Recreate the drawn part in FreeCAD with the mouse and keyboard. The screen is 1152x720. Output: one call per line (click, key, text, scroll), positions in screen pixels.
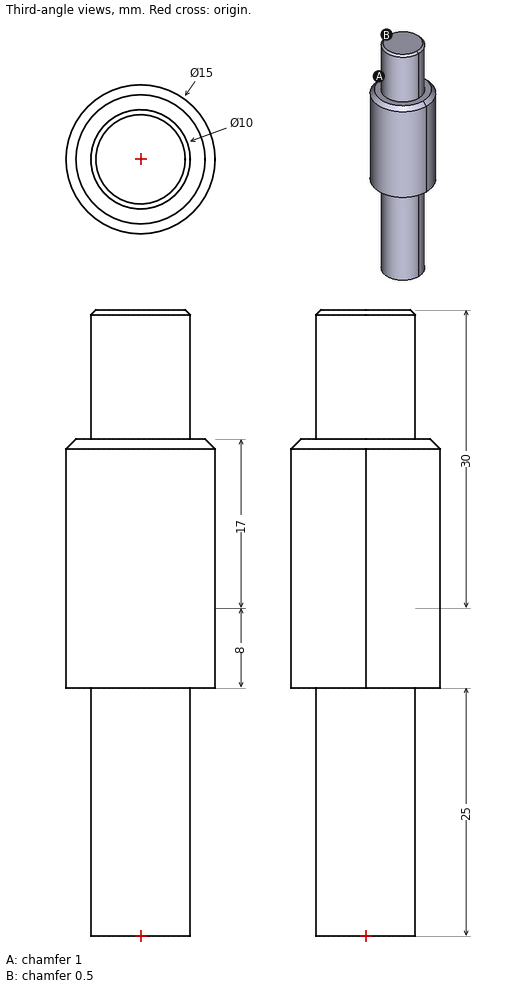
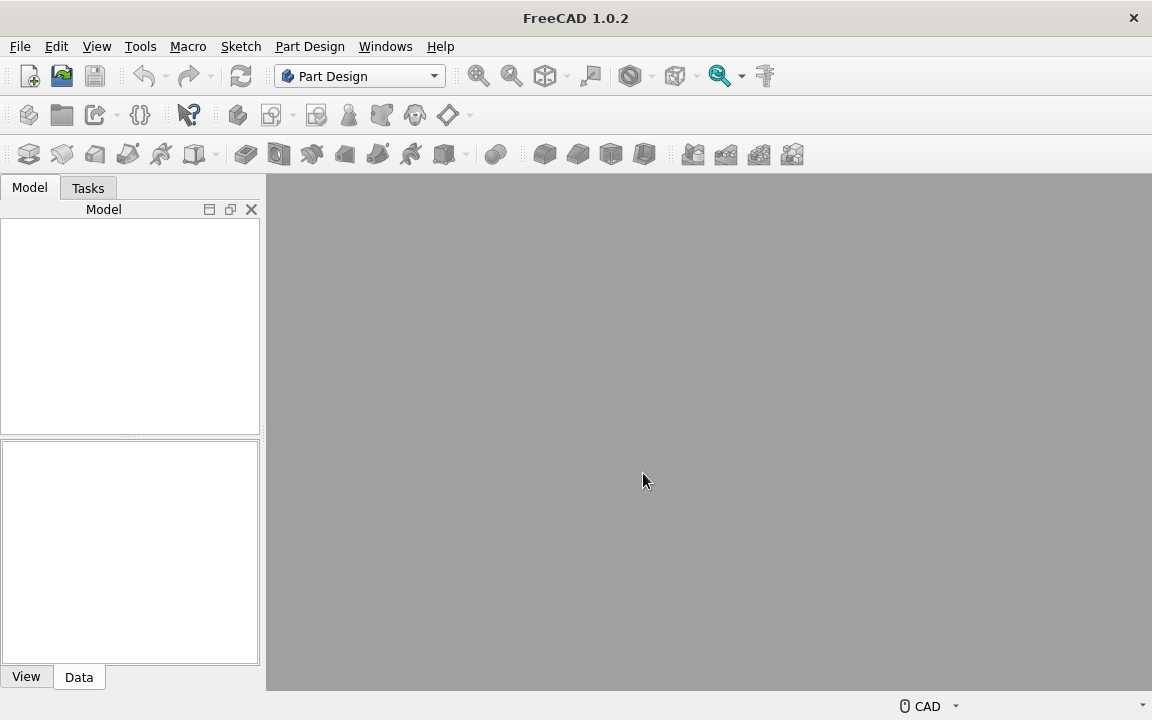
key(ctrl+n)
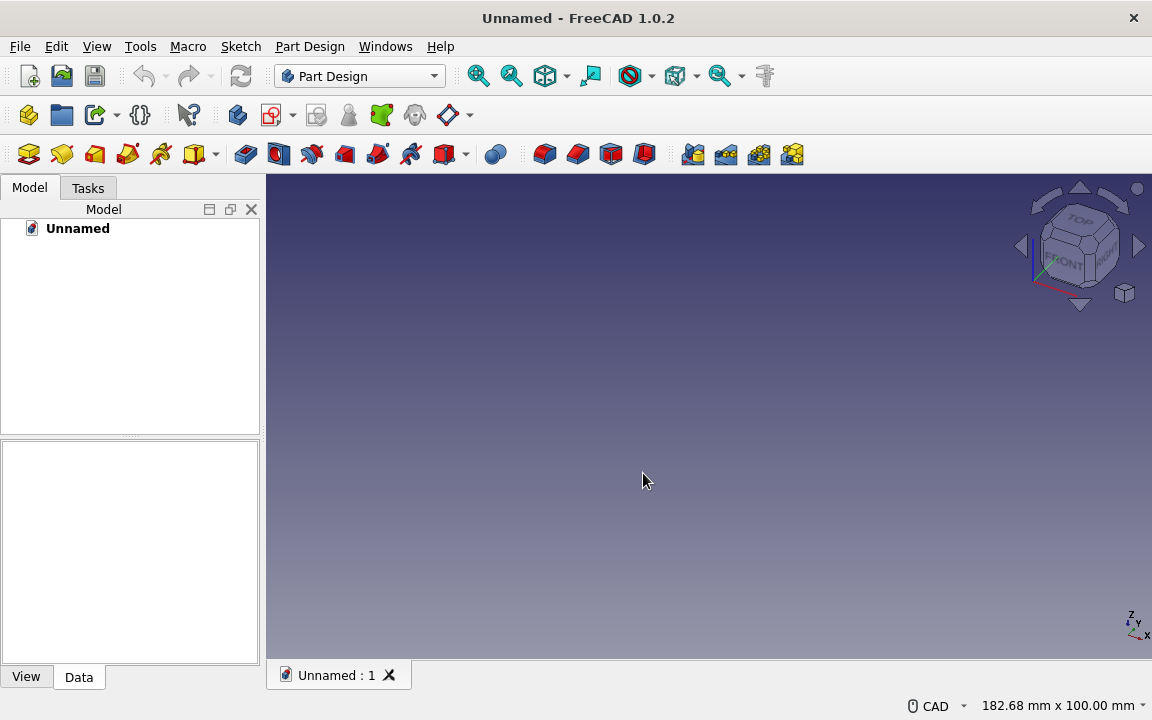
click(270, 116)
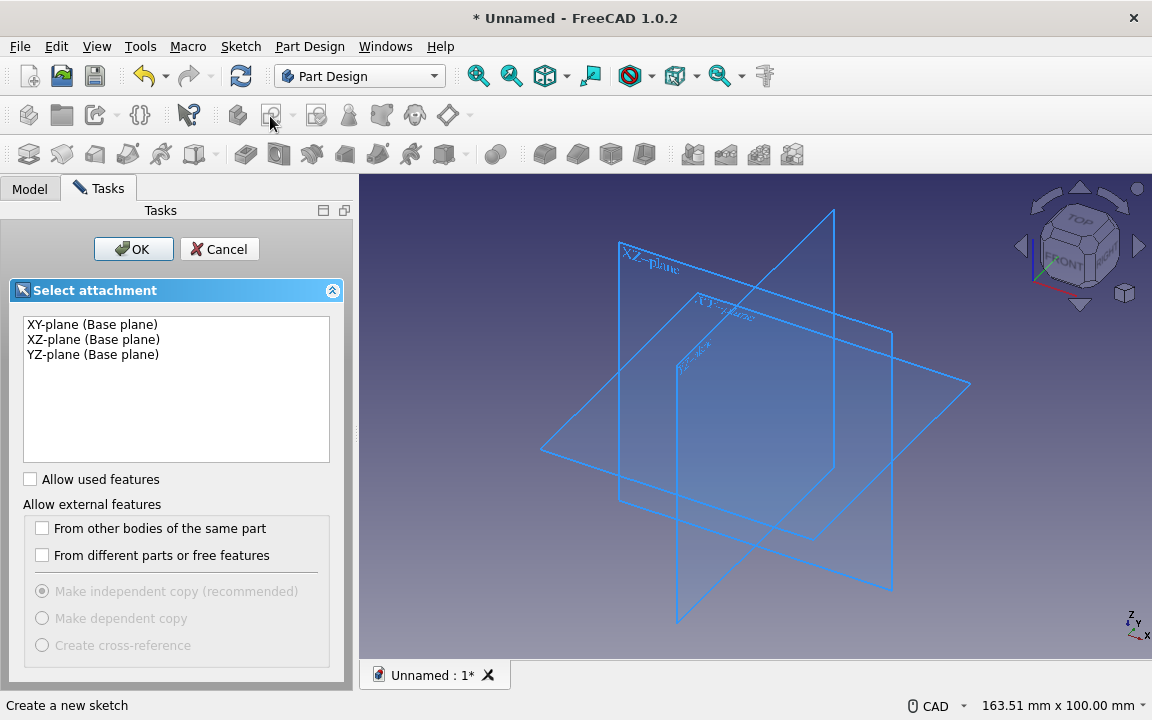
click(84, 324)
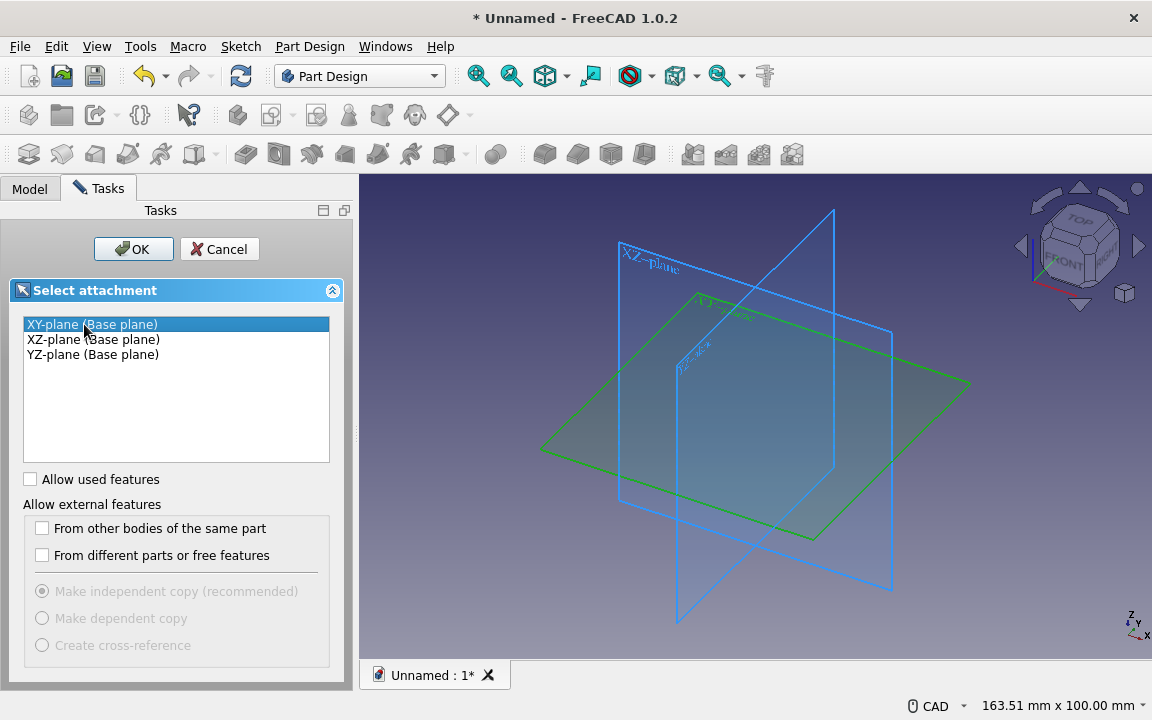
click(134, 249)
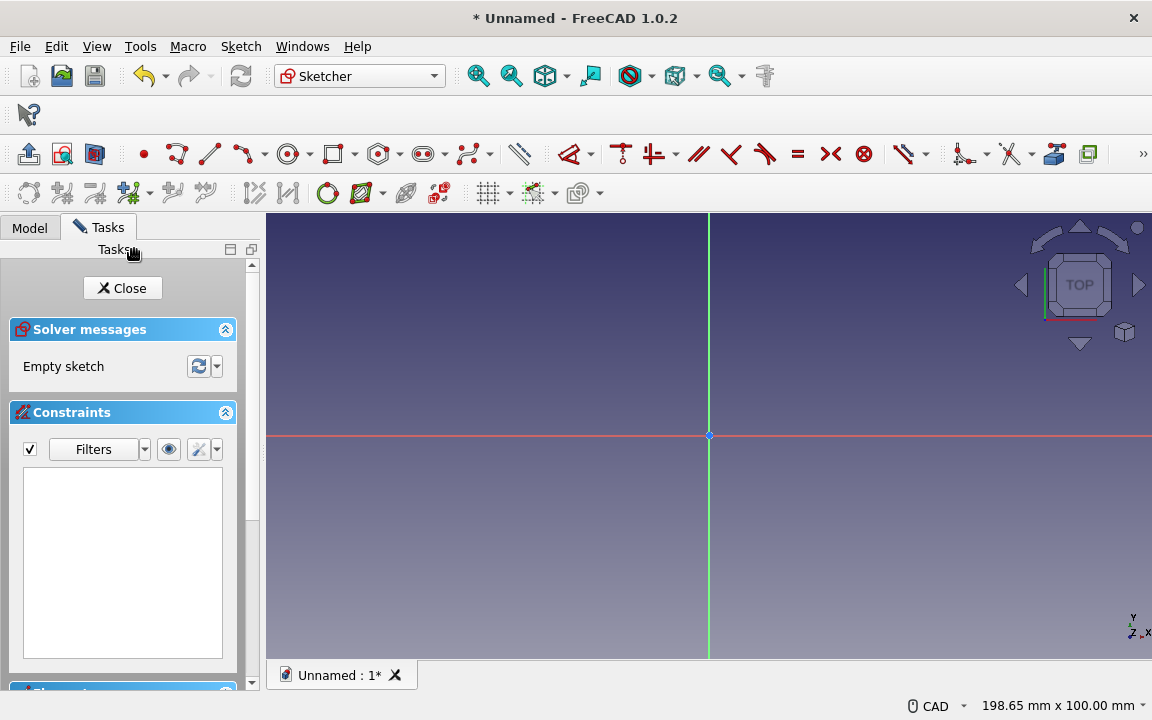
scroll(723, 436, up, 9)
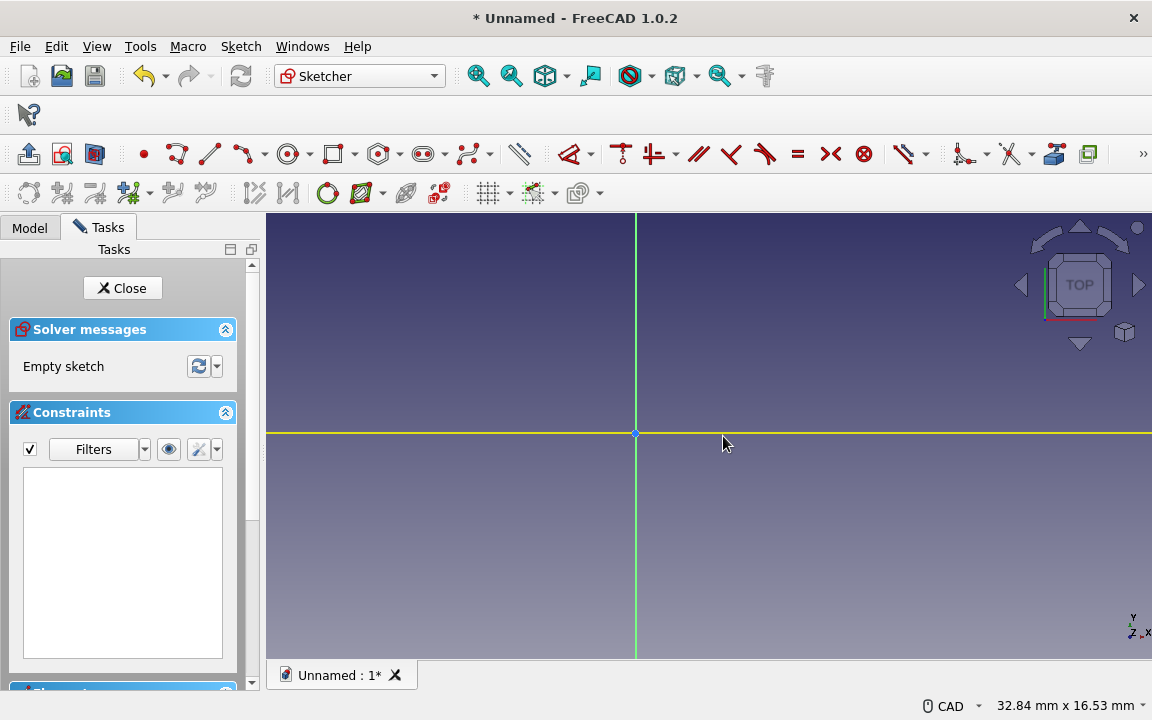
key(g)
key(c)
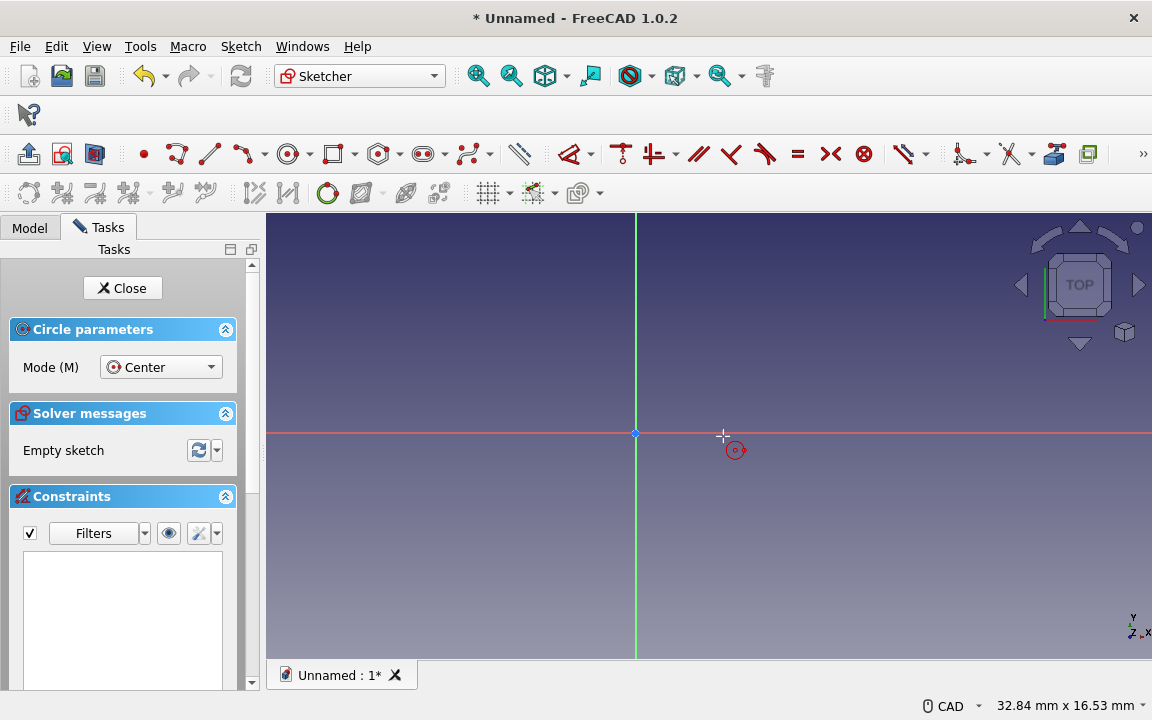
click(636, 433)
click(731, 338)
key(Escape)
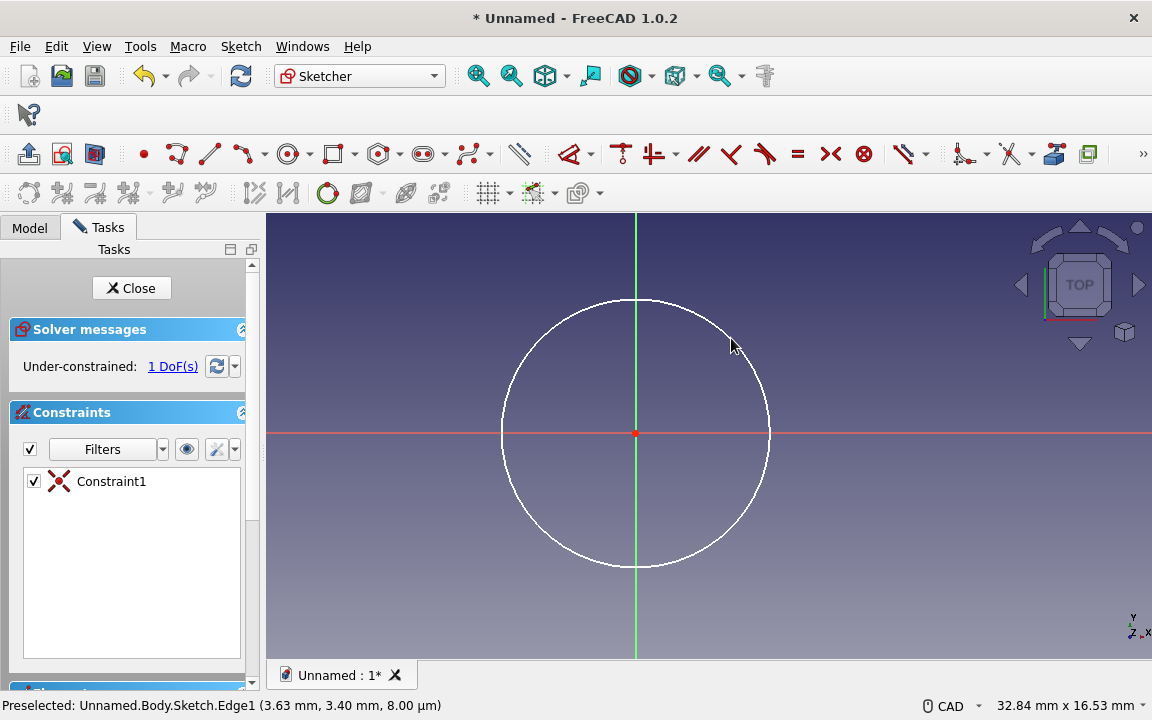
key(d)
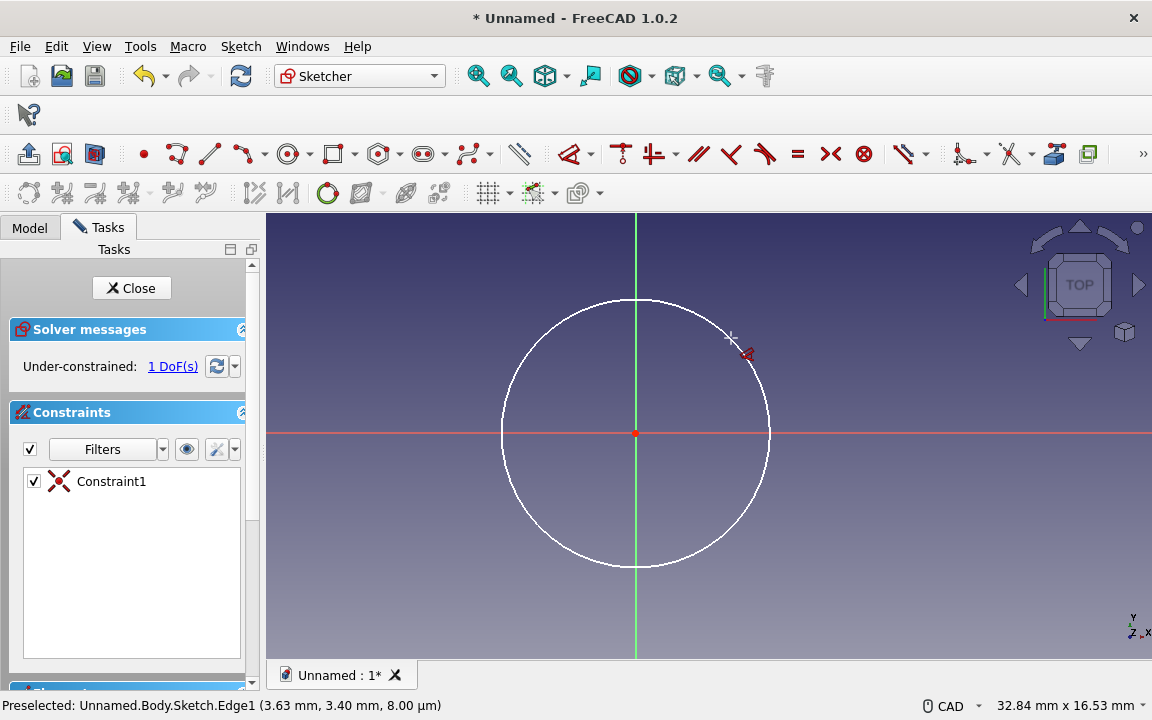
click(730, 338)
click(752, 315)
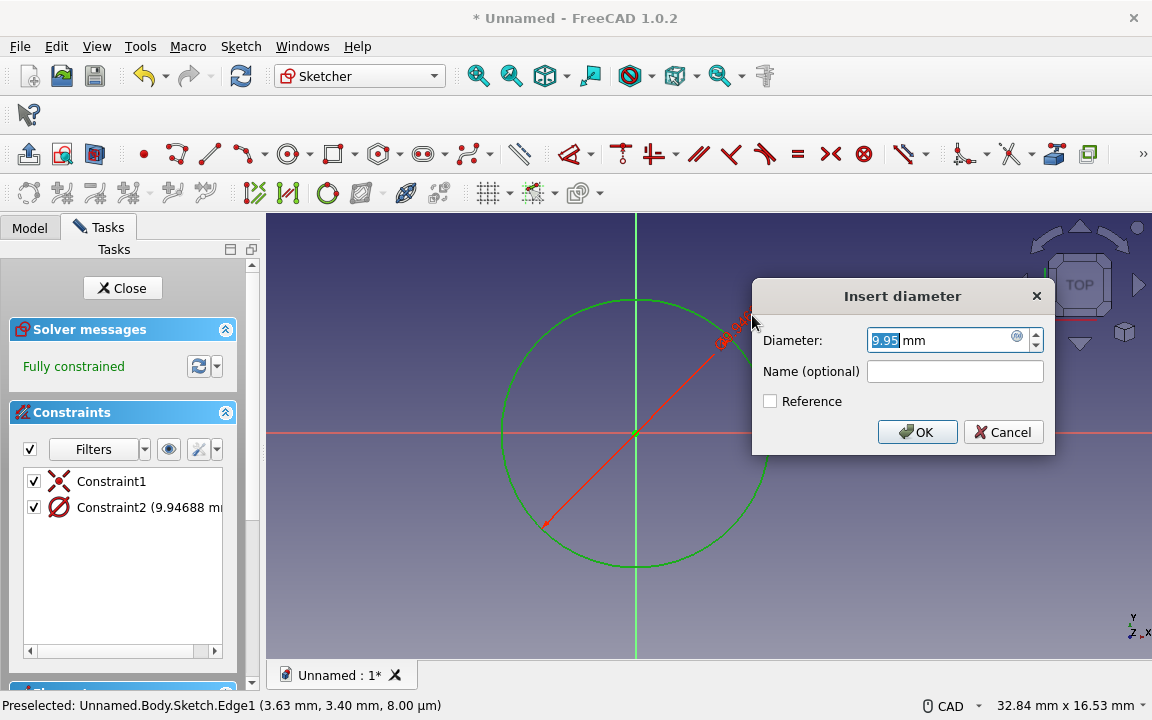
text(10)
key(Return)
key(Escape)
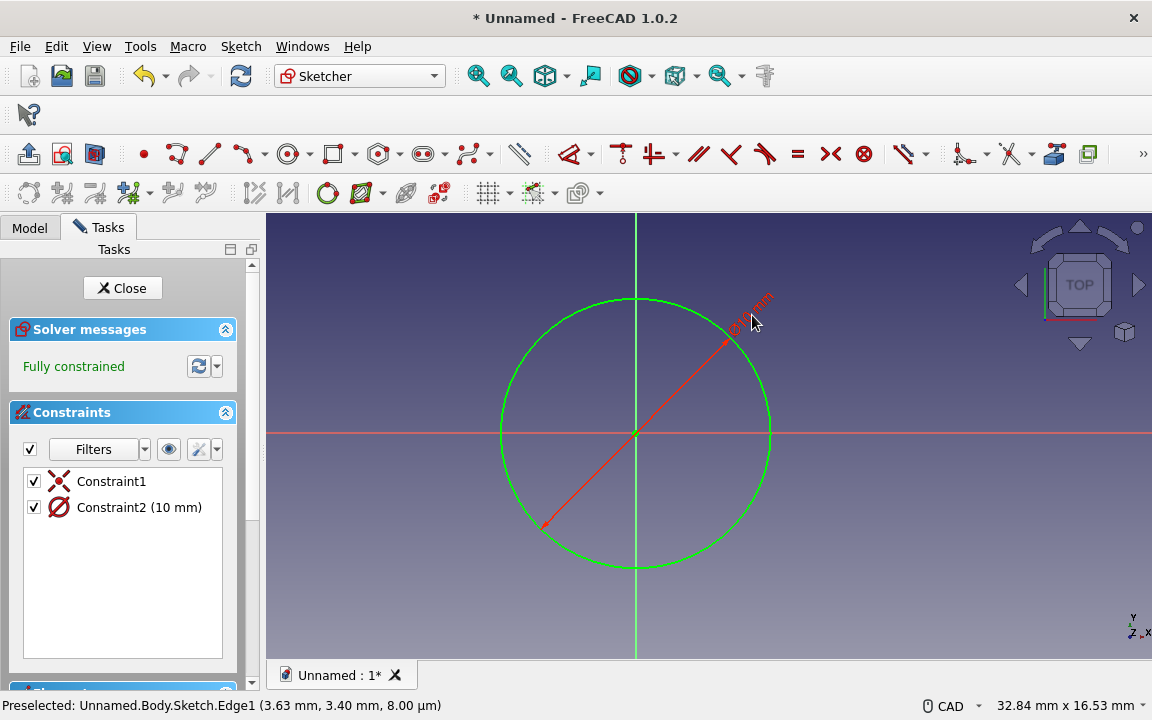
click(123, 288)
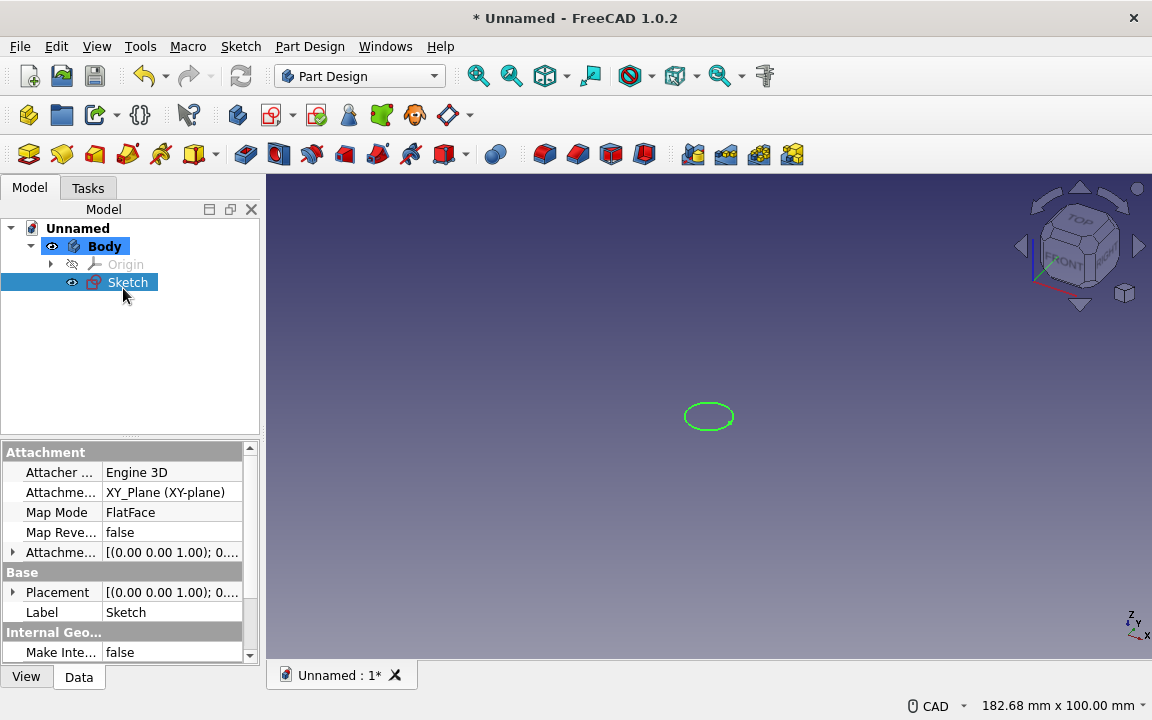
click(29, 154)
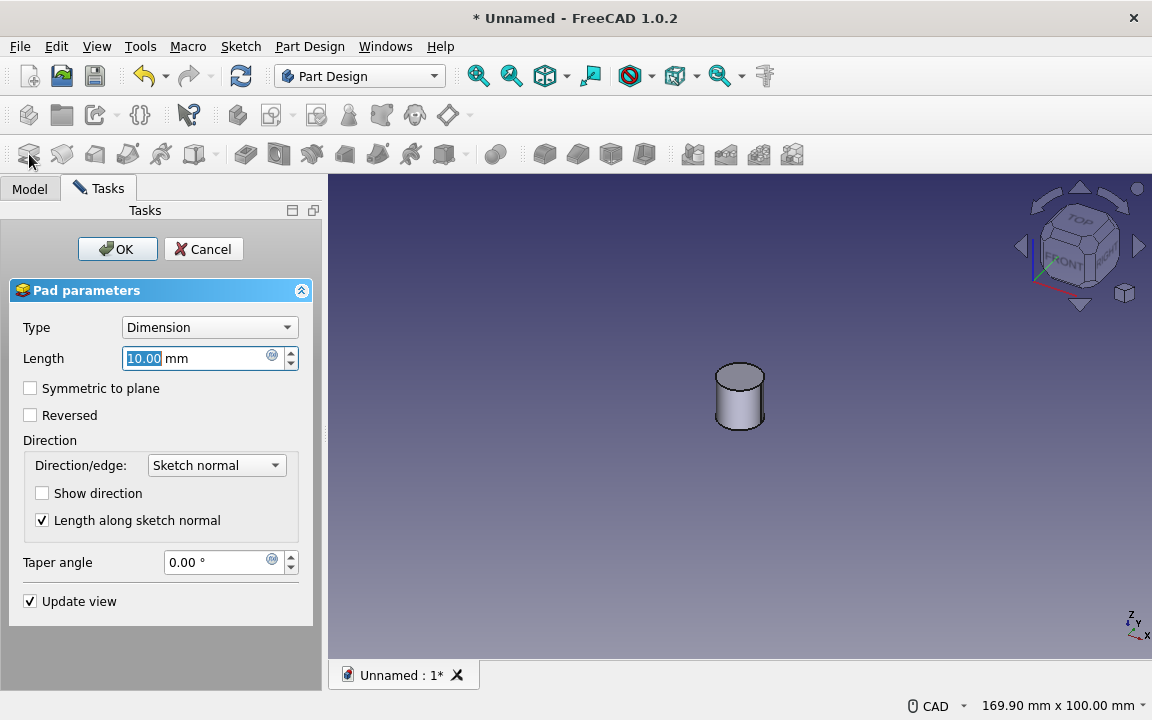
text(25)
key(Tab)